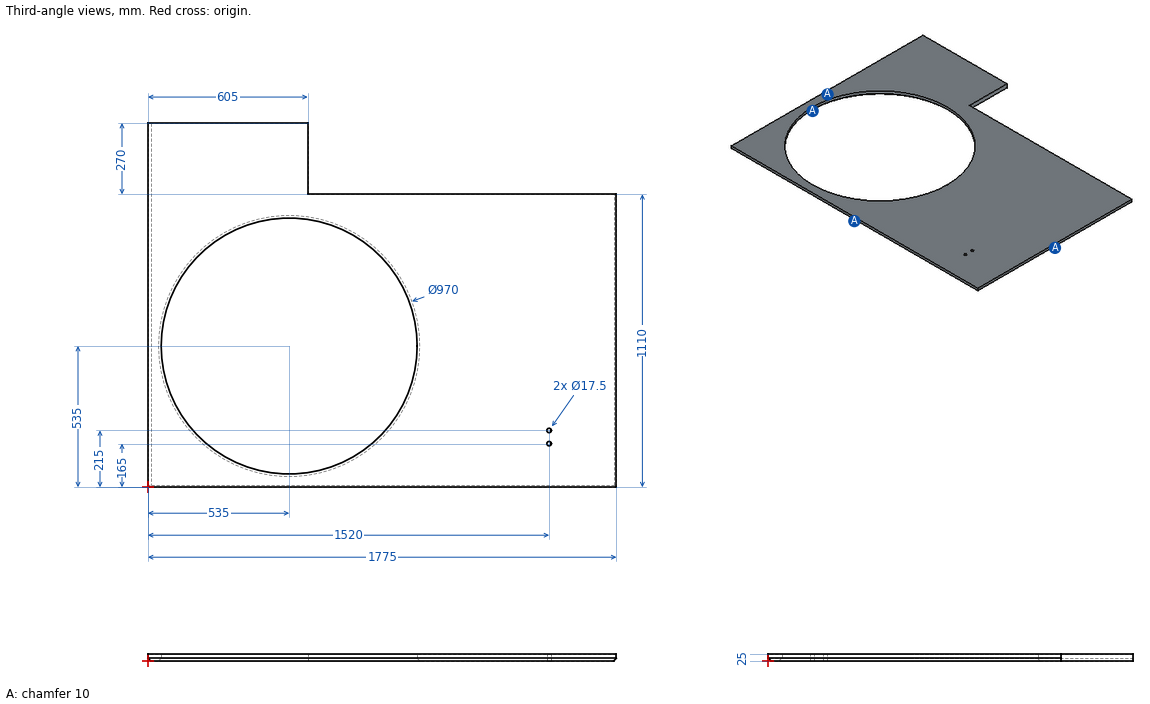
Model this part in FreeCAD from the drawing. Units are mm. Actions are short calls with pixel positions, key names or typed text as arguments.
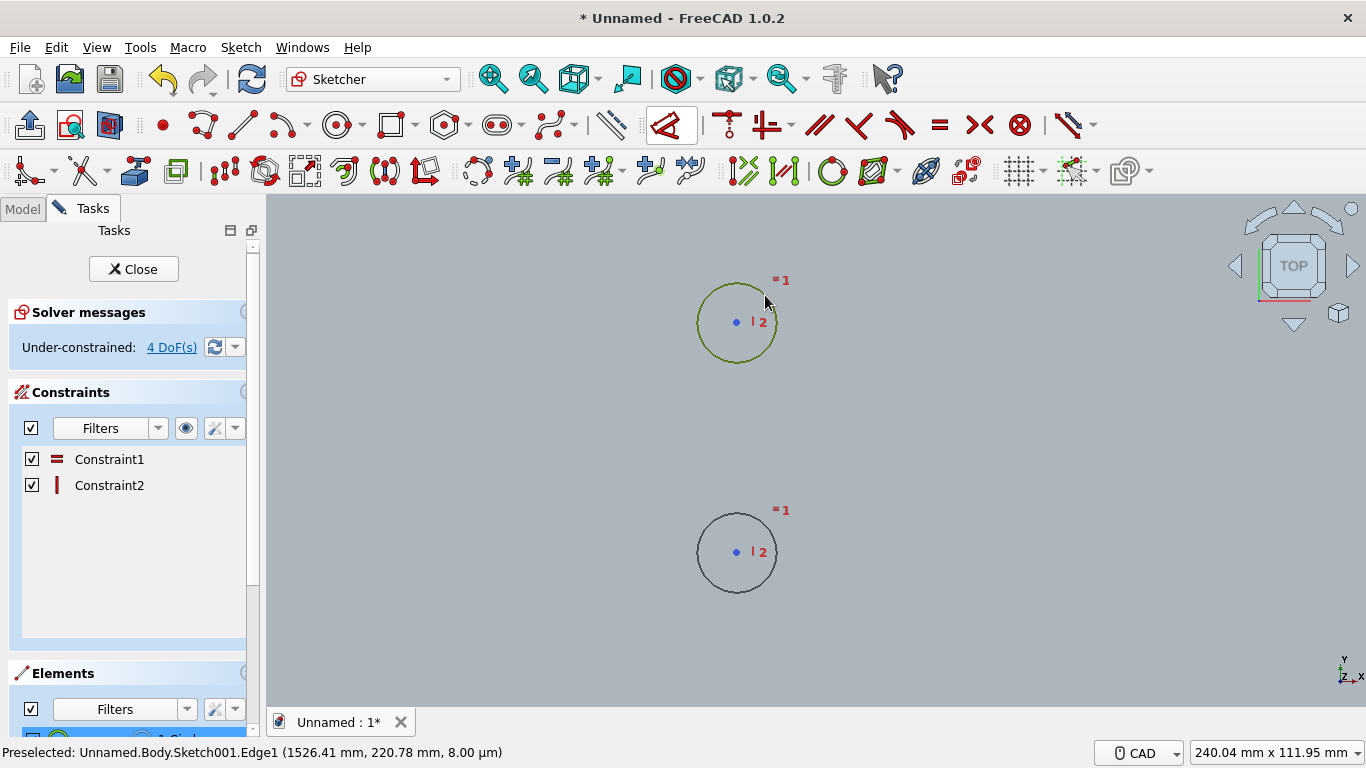
click(692, 126)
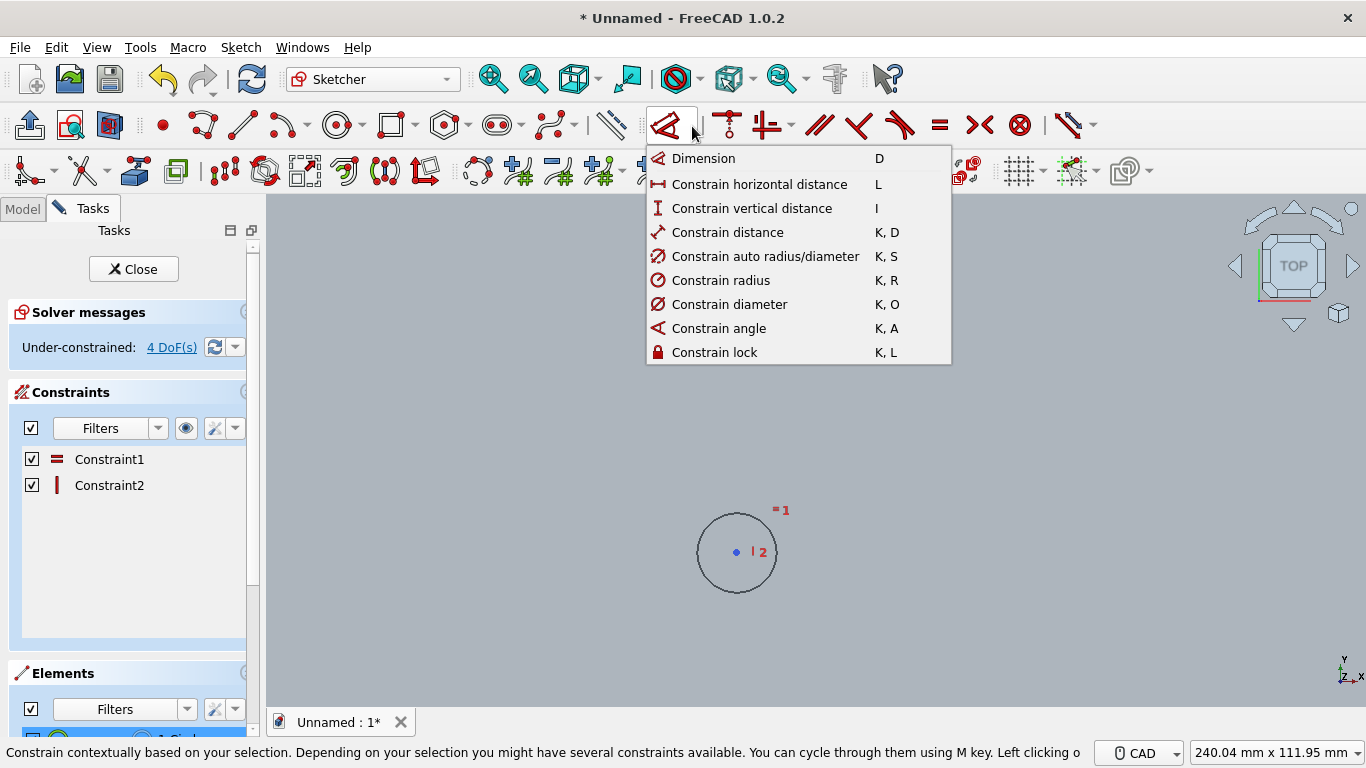
click(799, 304)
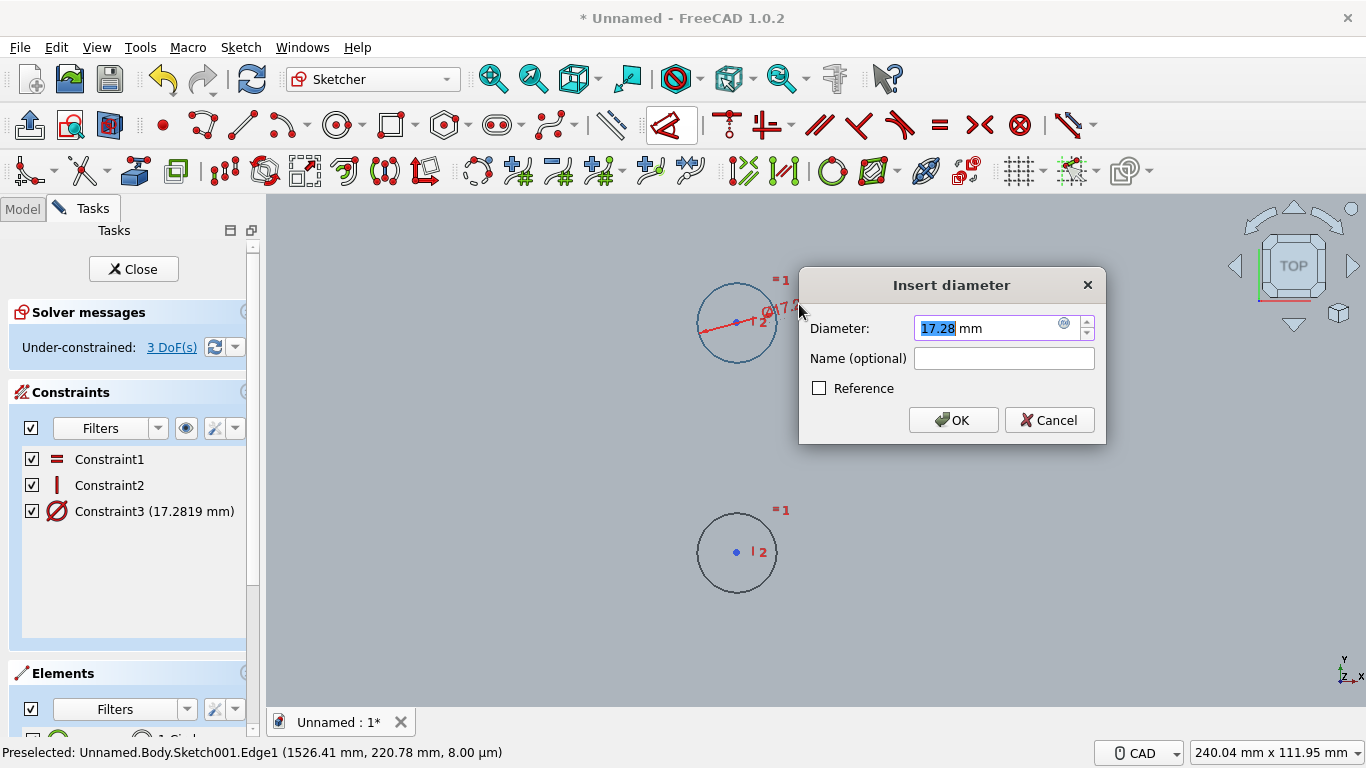
text(17.5)
key(Return)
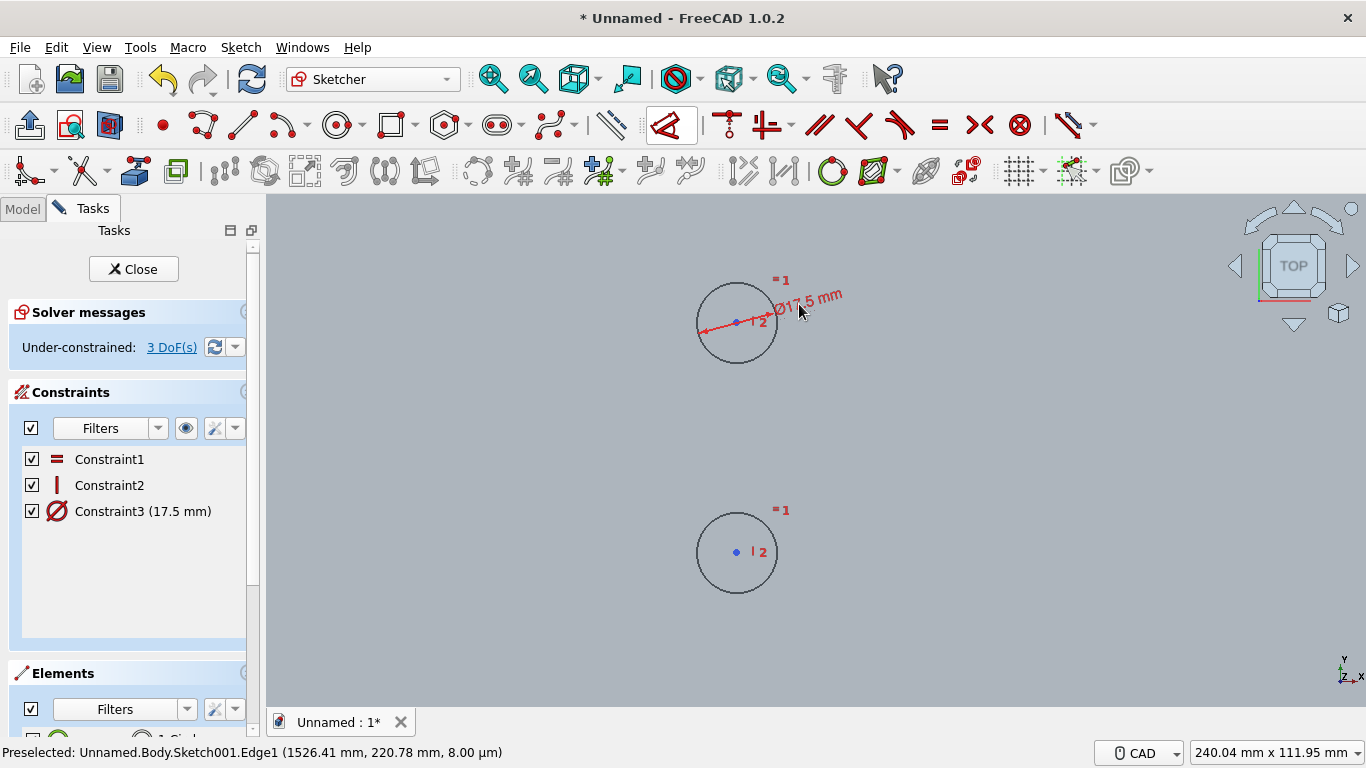
click(737, 323)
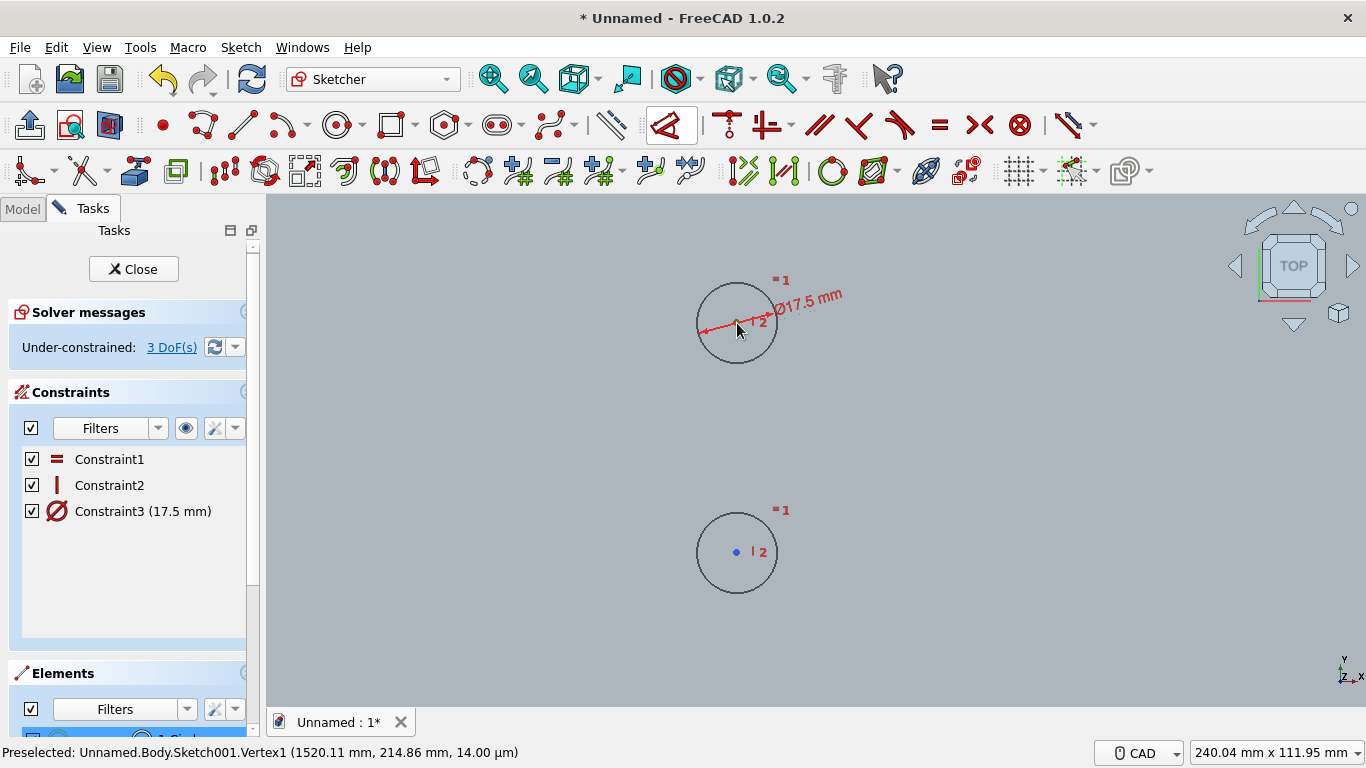
click(692, 126)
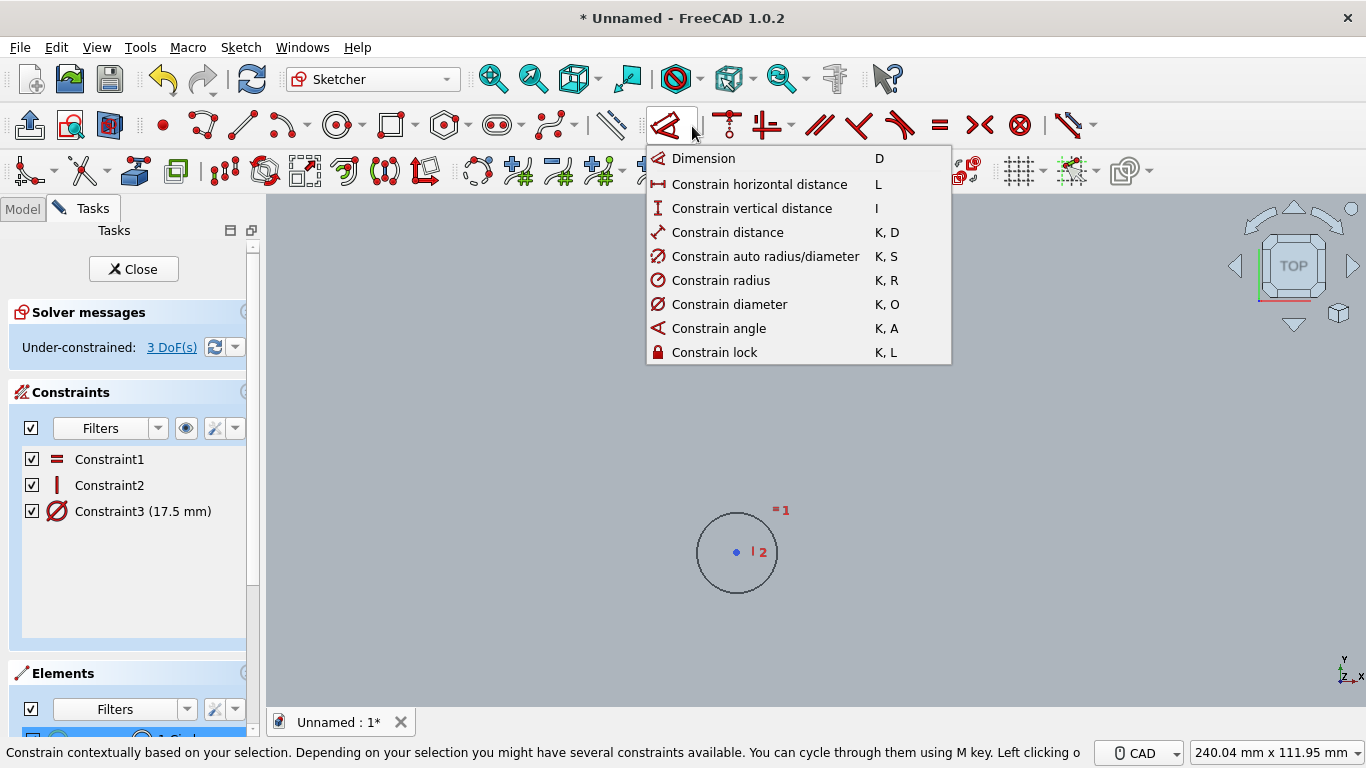
click(799, 208)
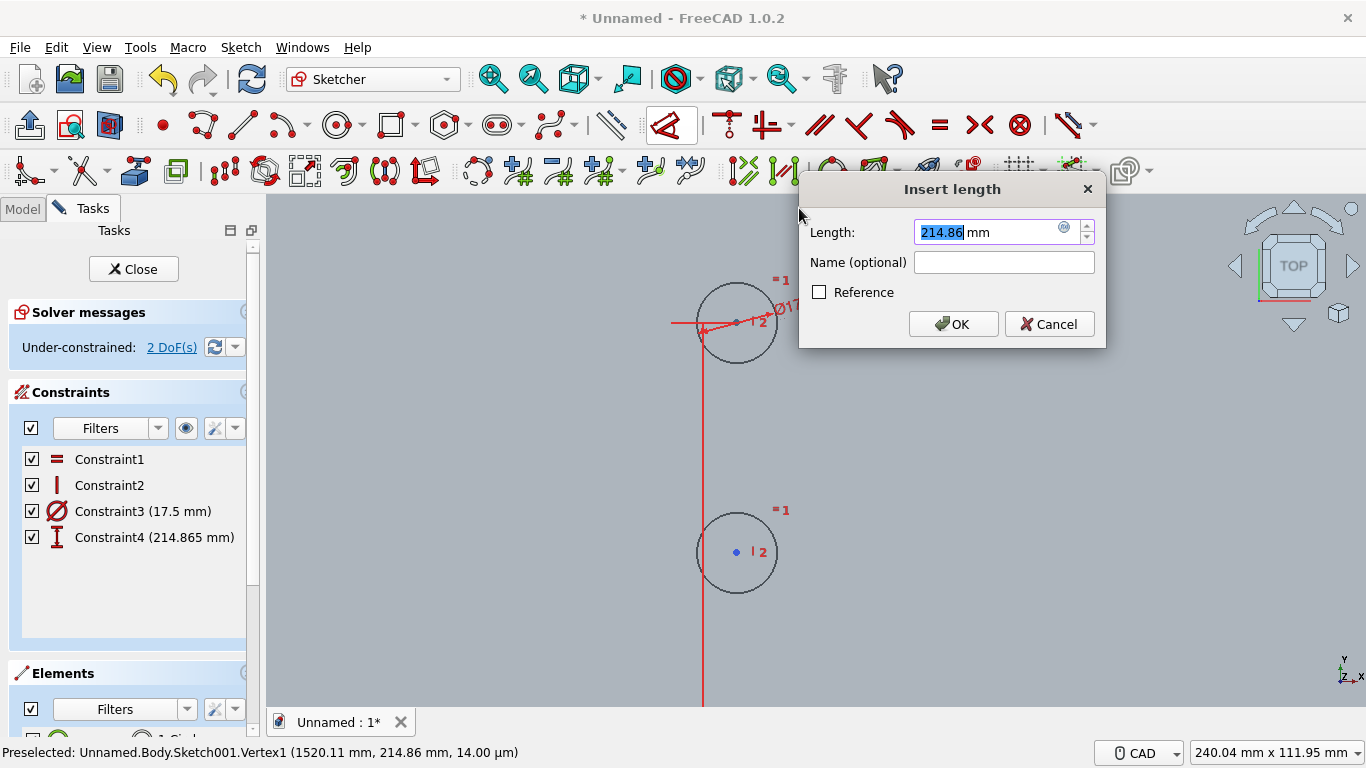
text(215)
key(Return)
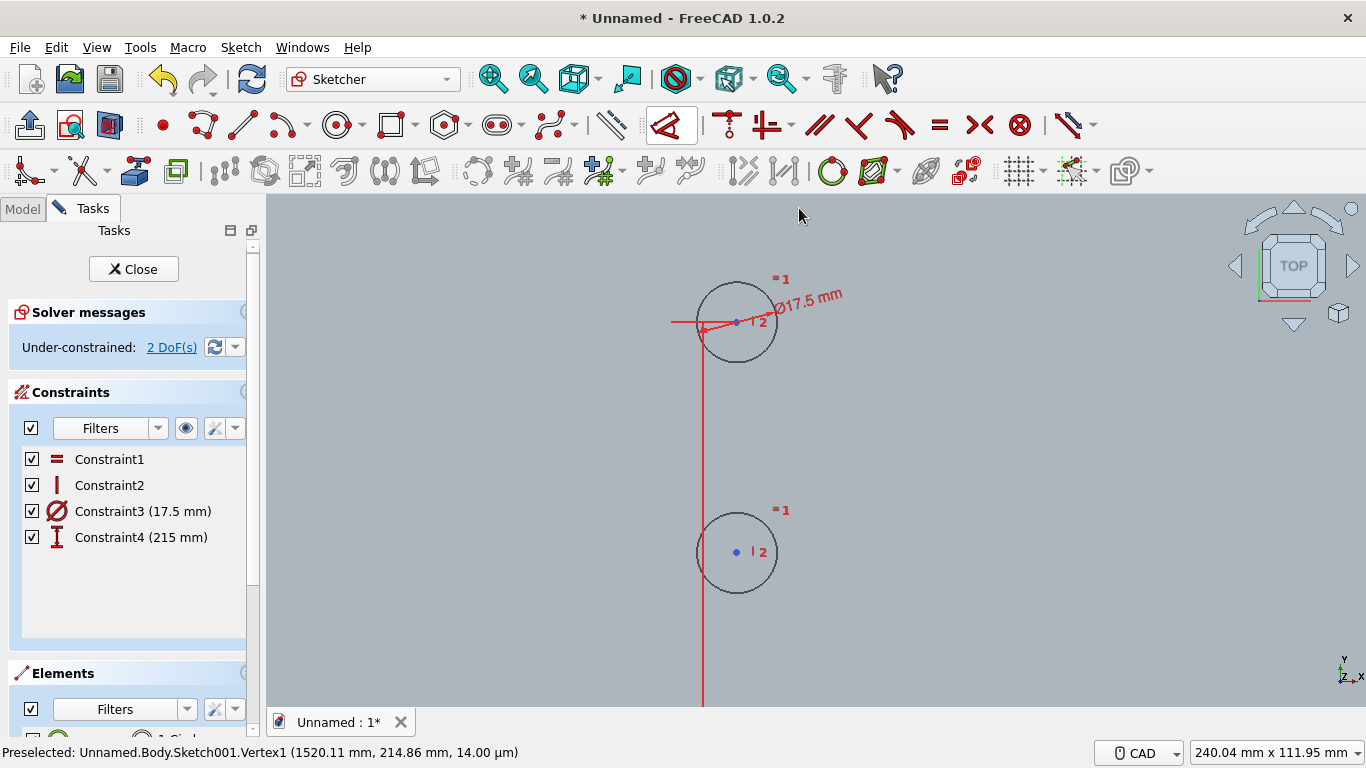
click(737, 553)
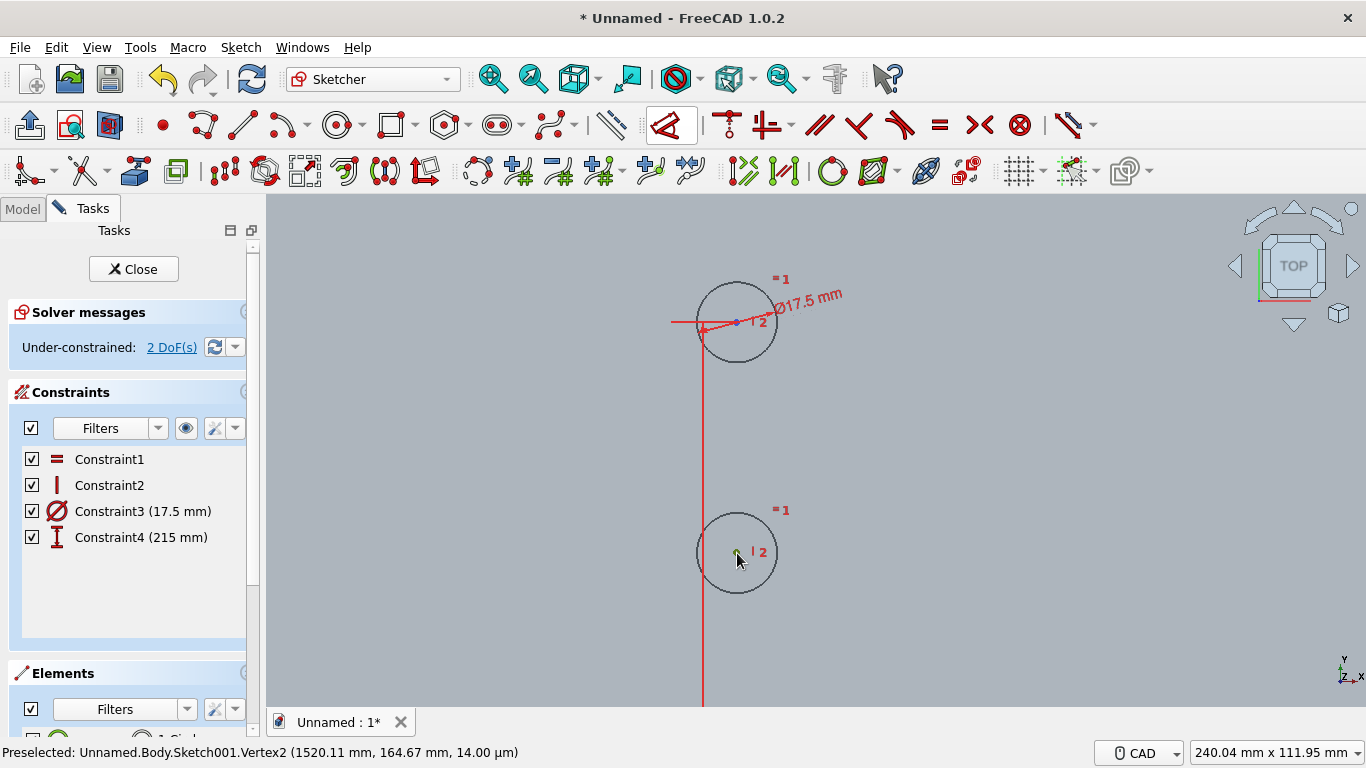
click(692, 126)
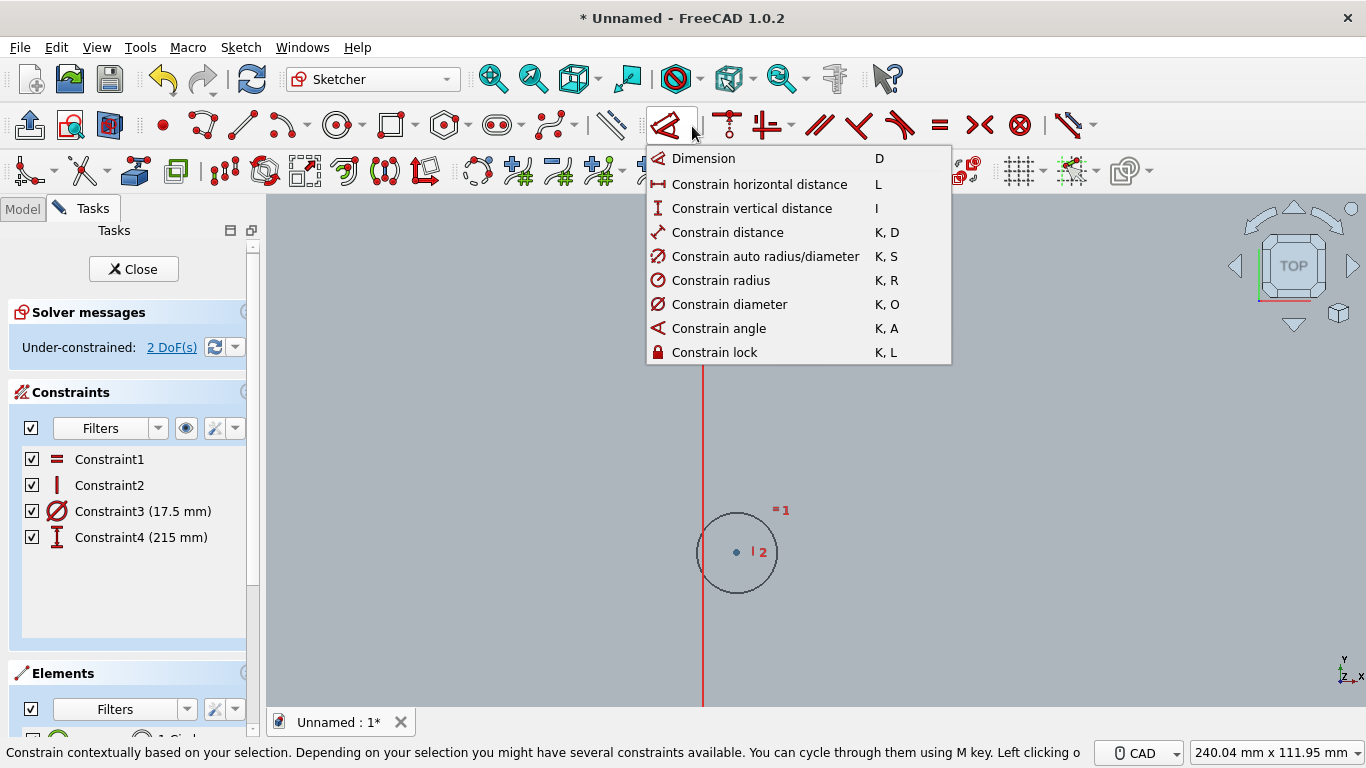
click(799, 208)